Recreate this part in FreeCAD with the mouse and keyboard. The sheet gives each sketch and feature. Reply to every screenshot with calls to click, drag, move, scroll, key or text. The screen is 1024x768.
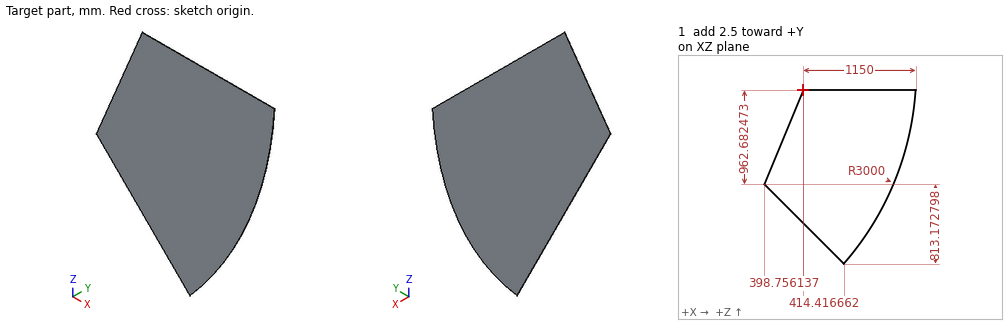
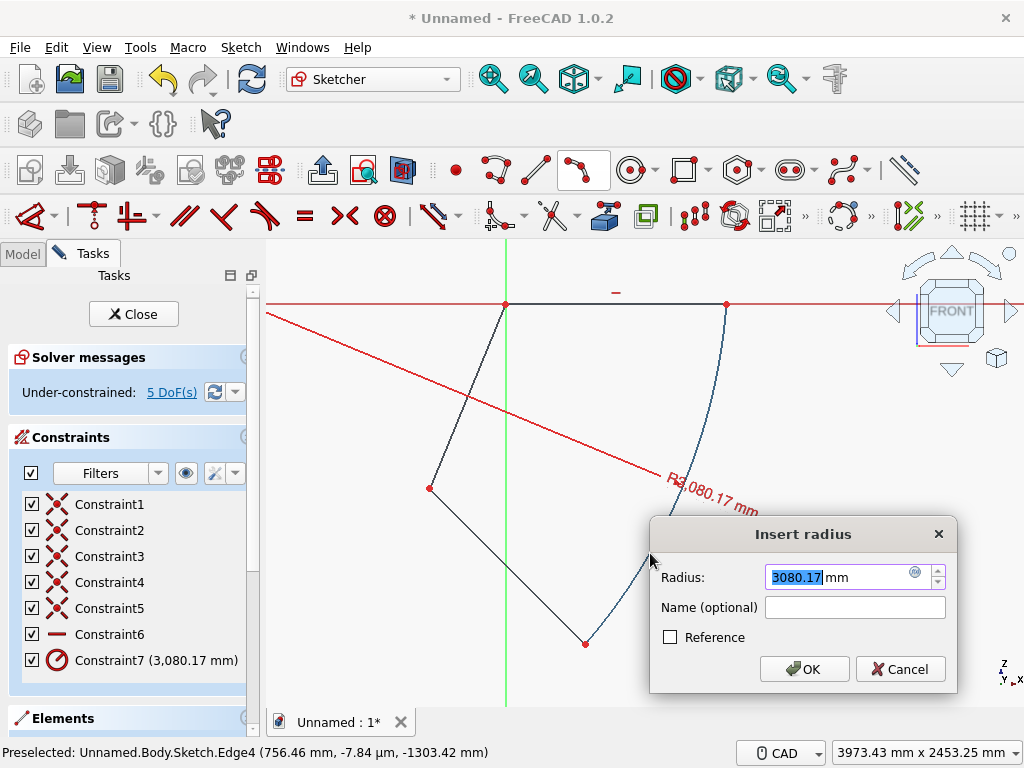
text(3000)
key(Return)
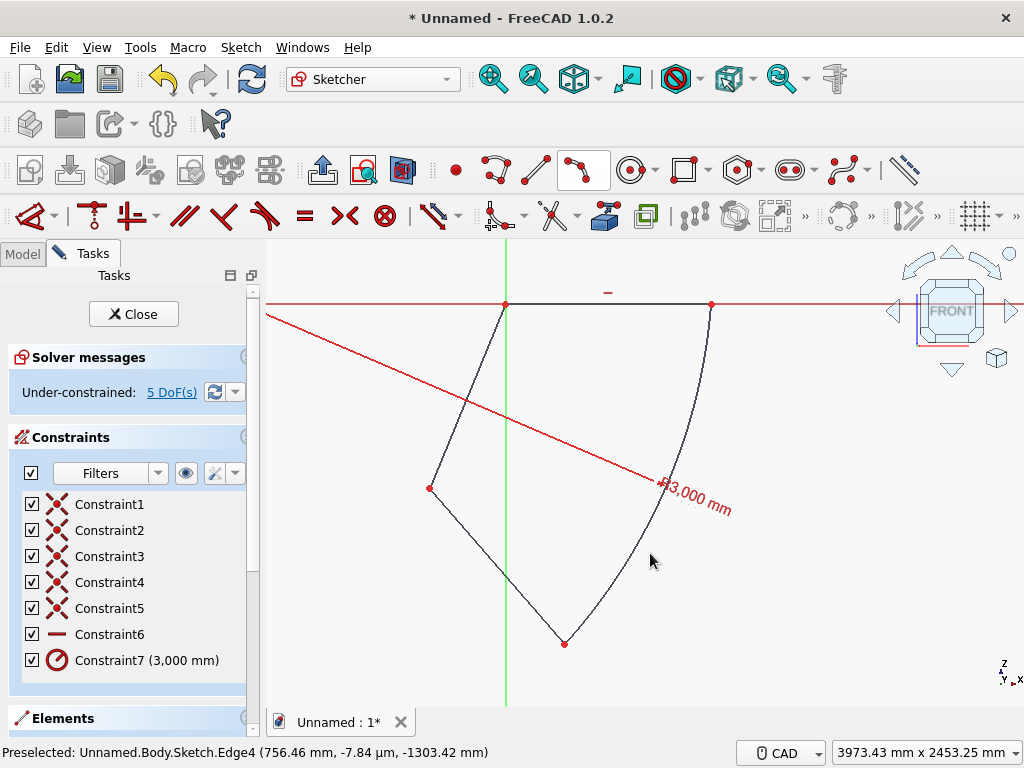
click(567, 304)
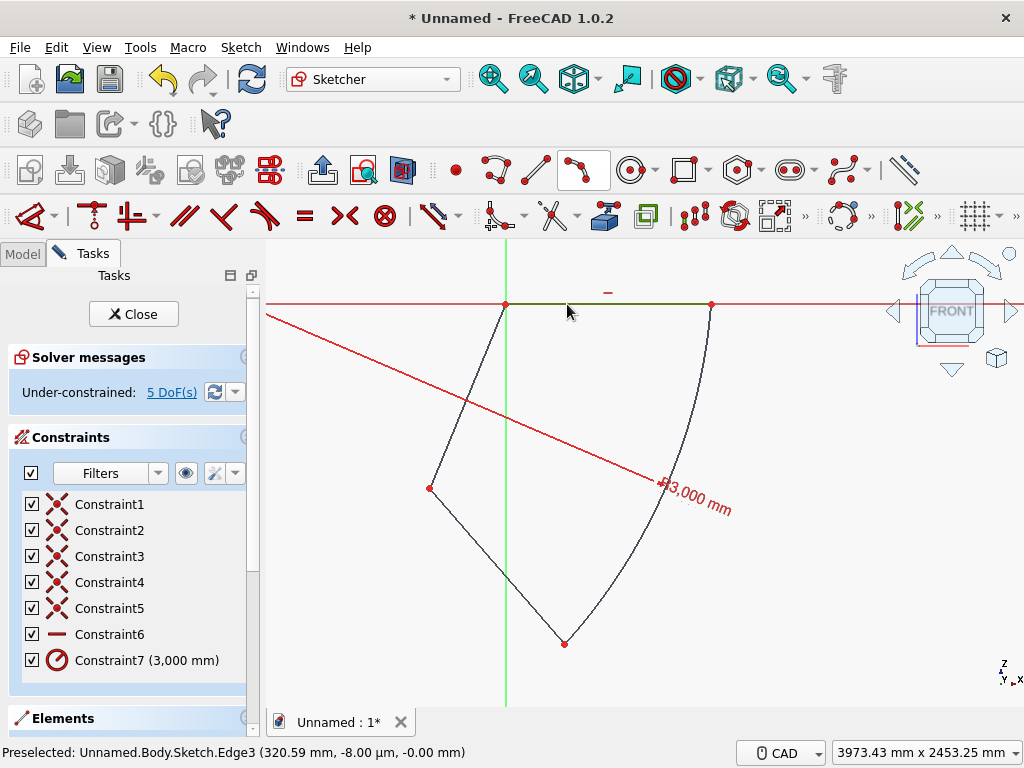
key(l)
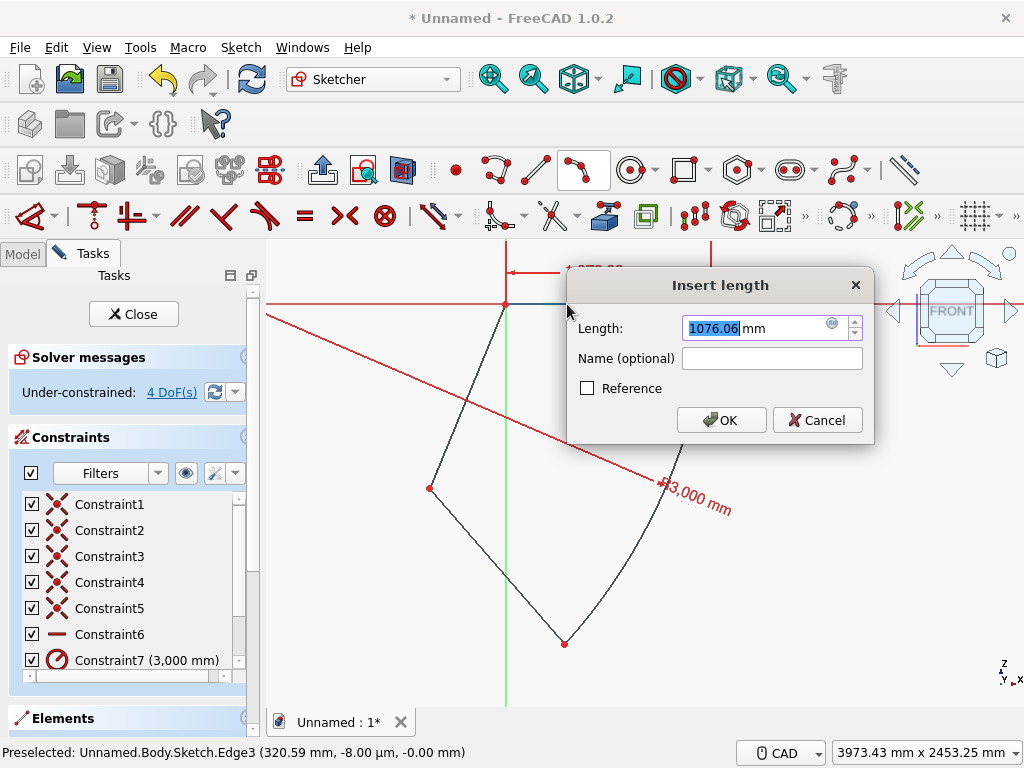
text(1150)
key(Return)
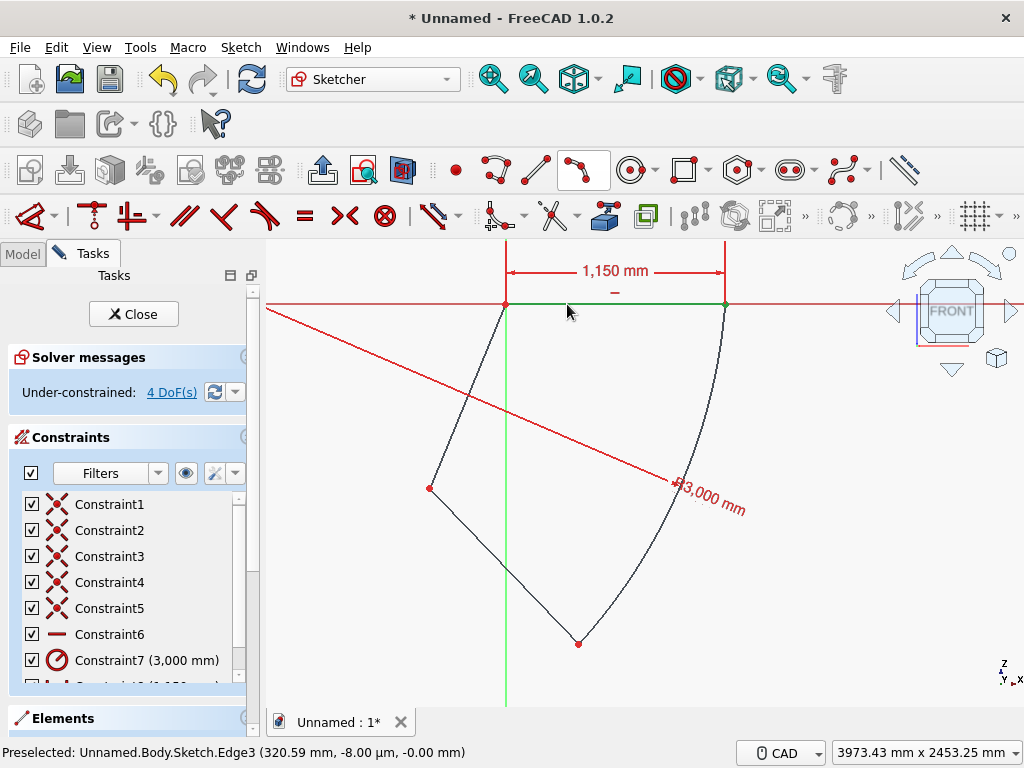
click(579, 644)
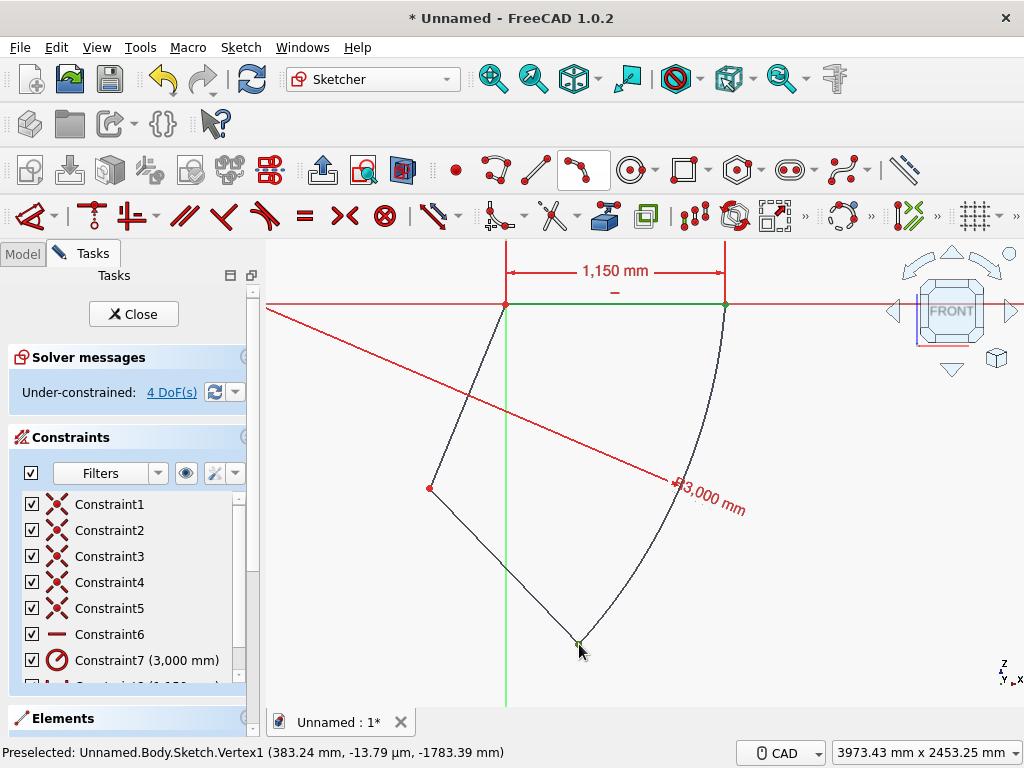
key(l)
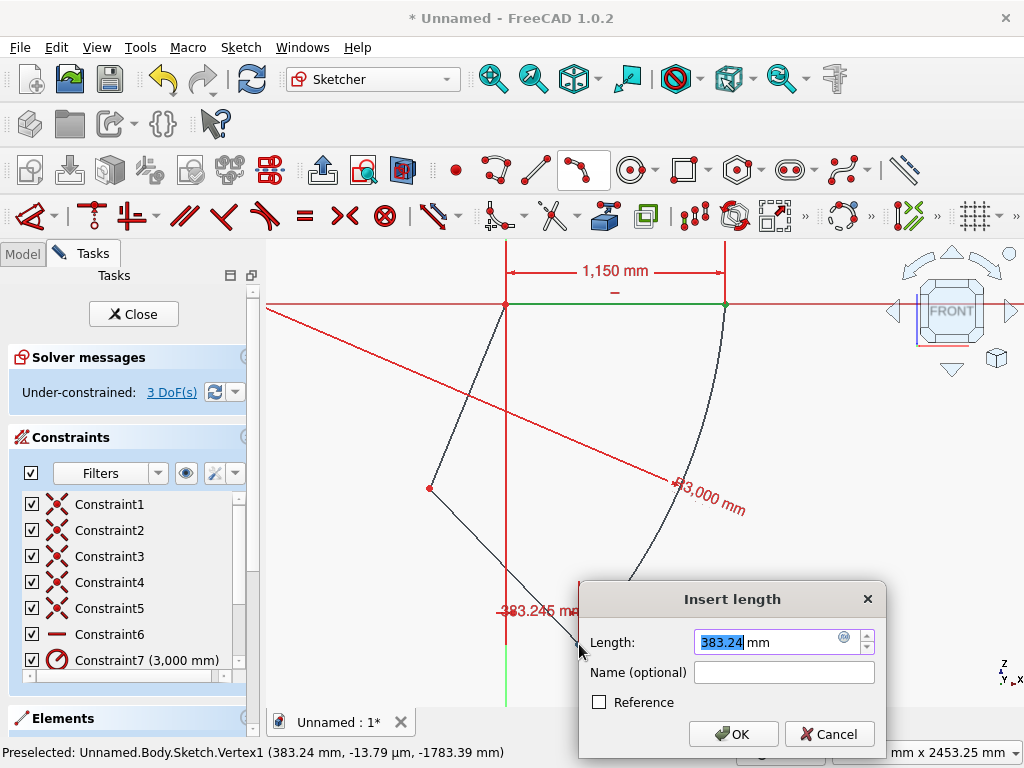
text(414.416662)
key(Return)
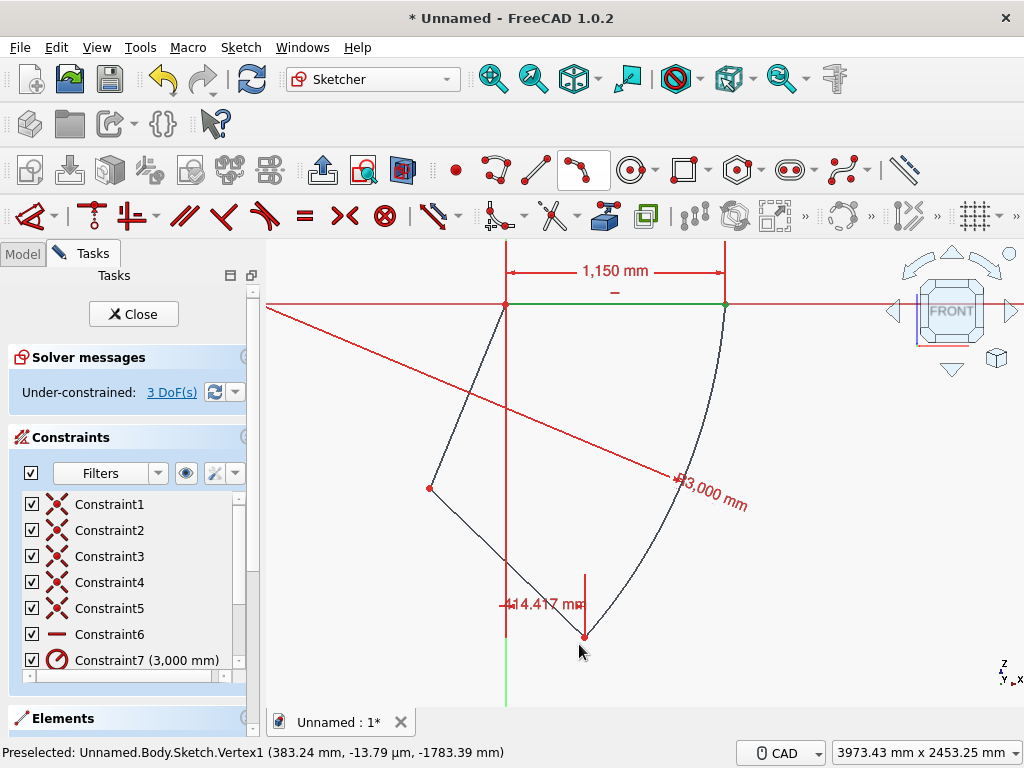
click(430, 489)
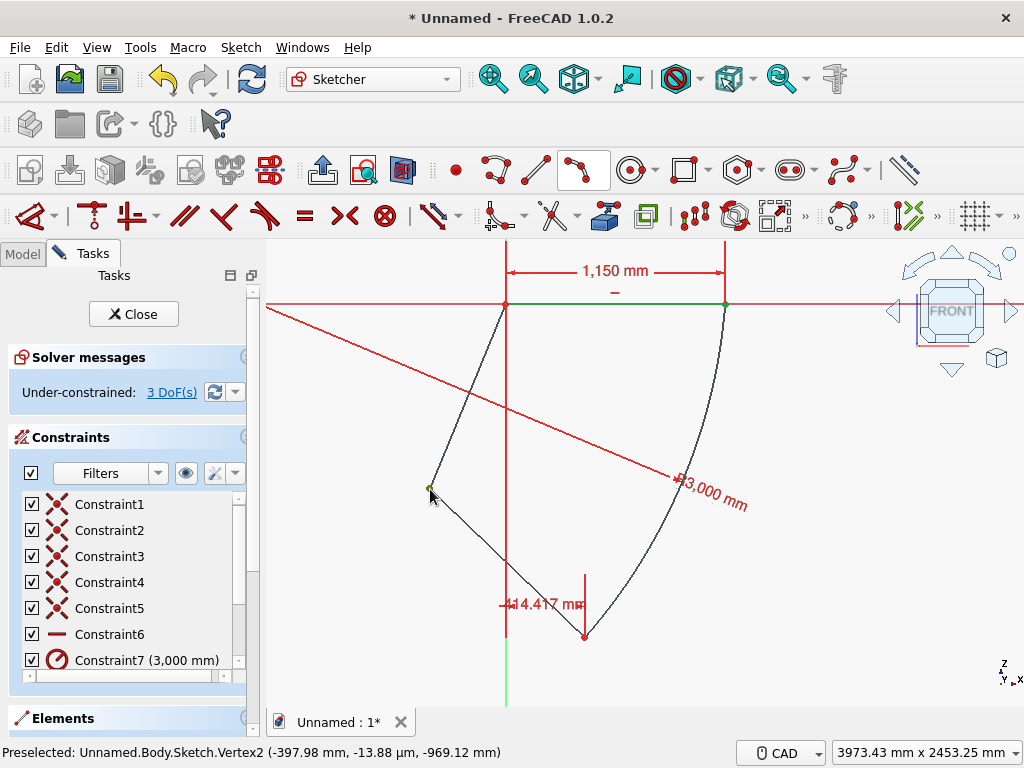
click(56, 216)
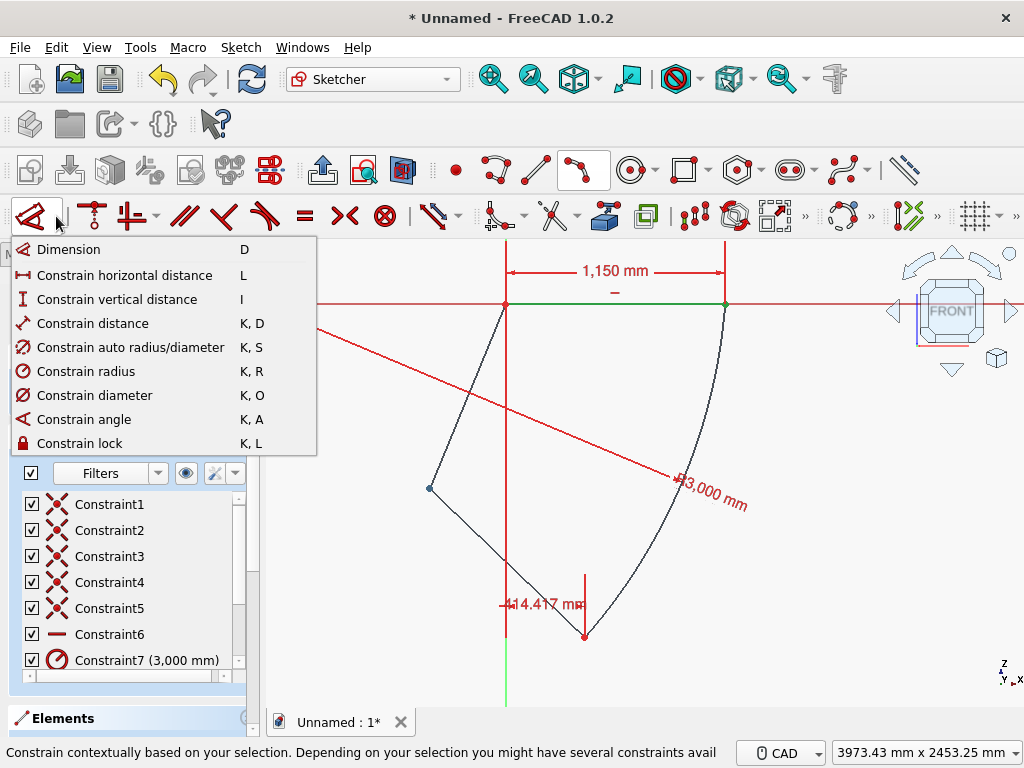
click(164, 275)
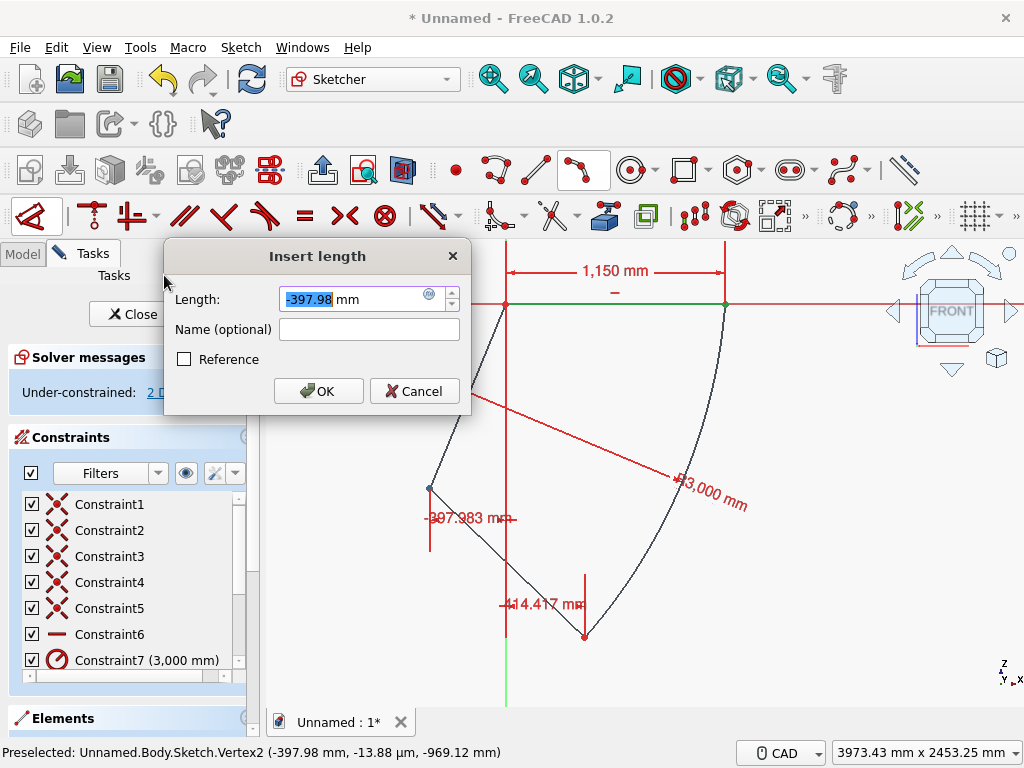
text(-398.756137)
key(Return)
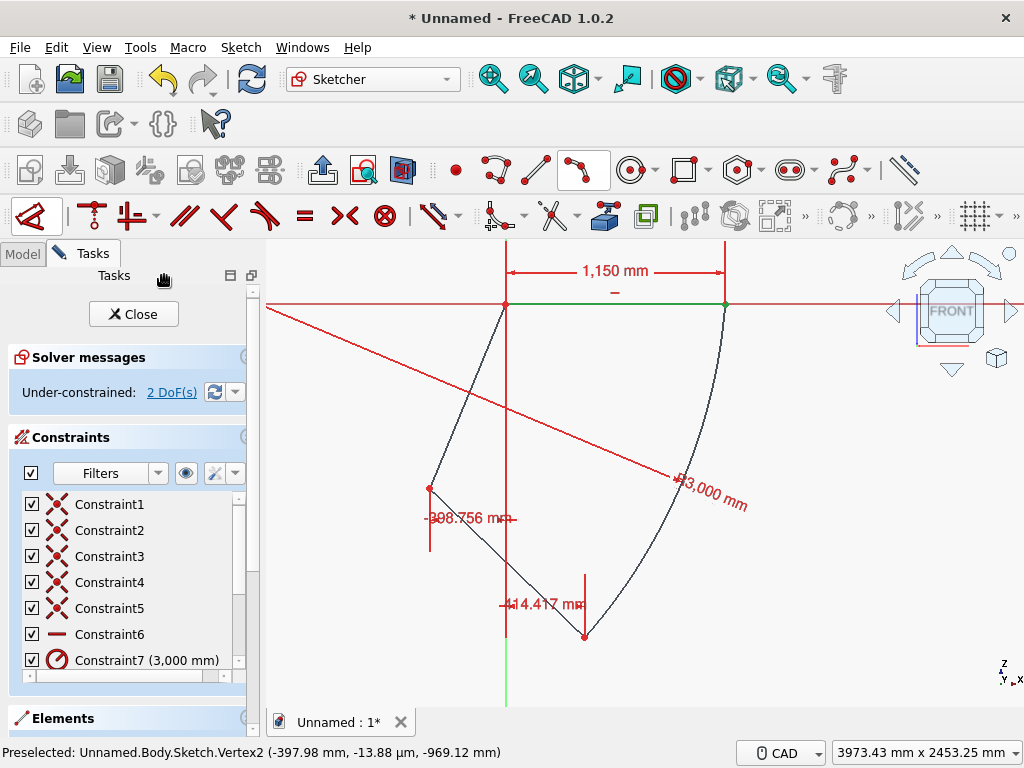
click(430, 489)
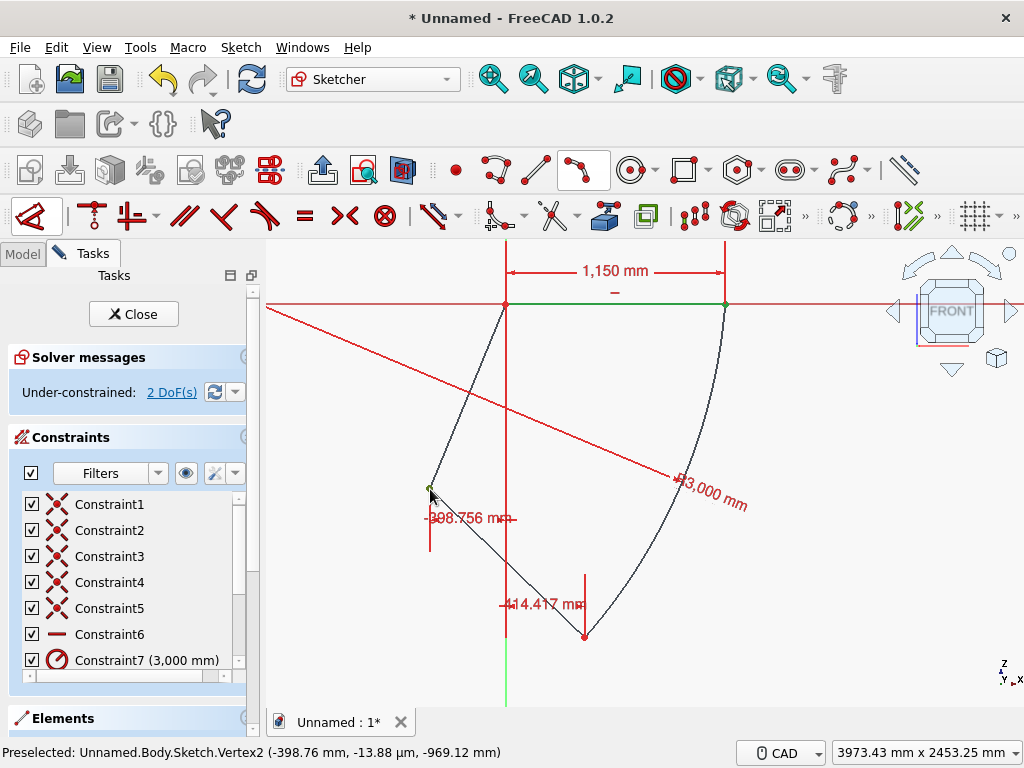
key(i)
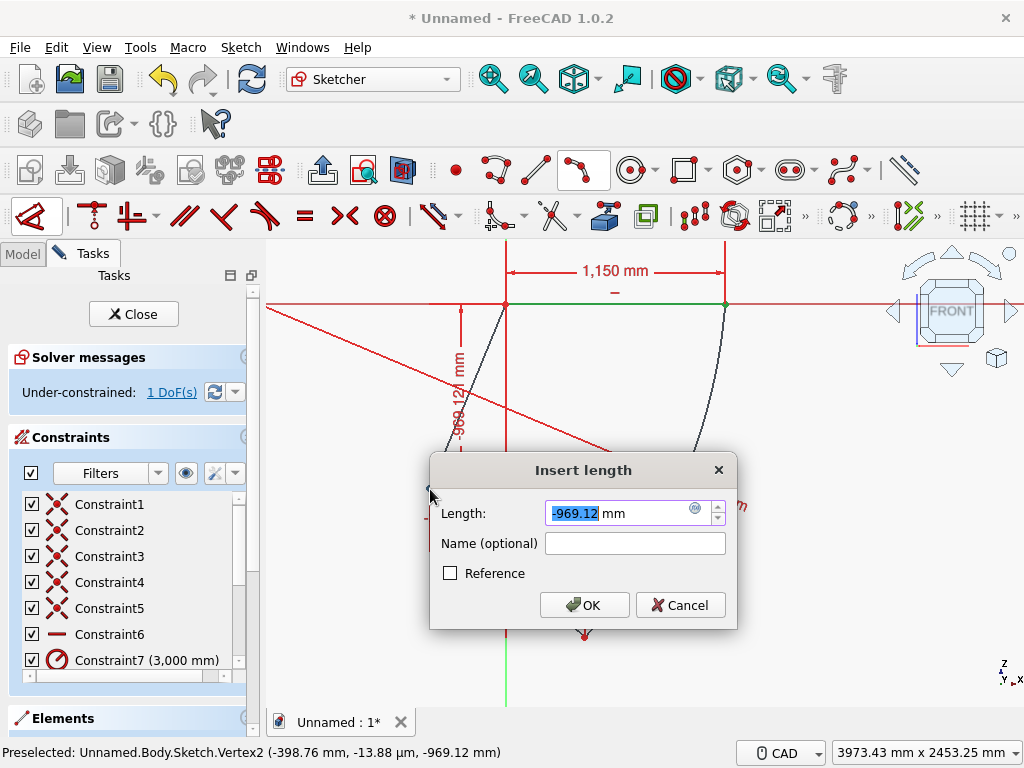
text(-962.682473)
key(Return)